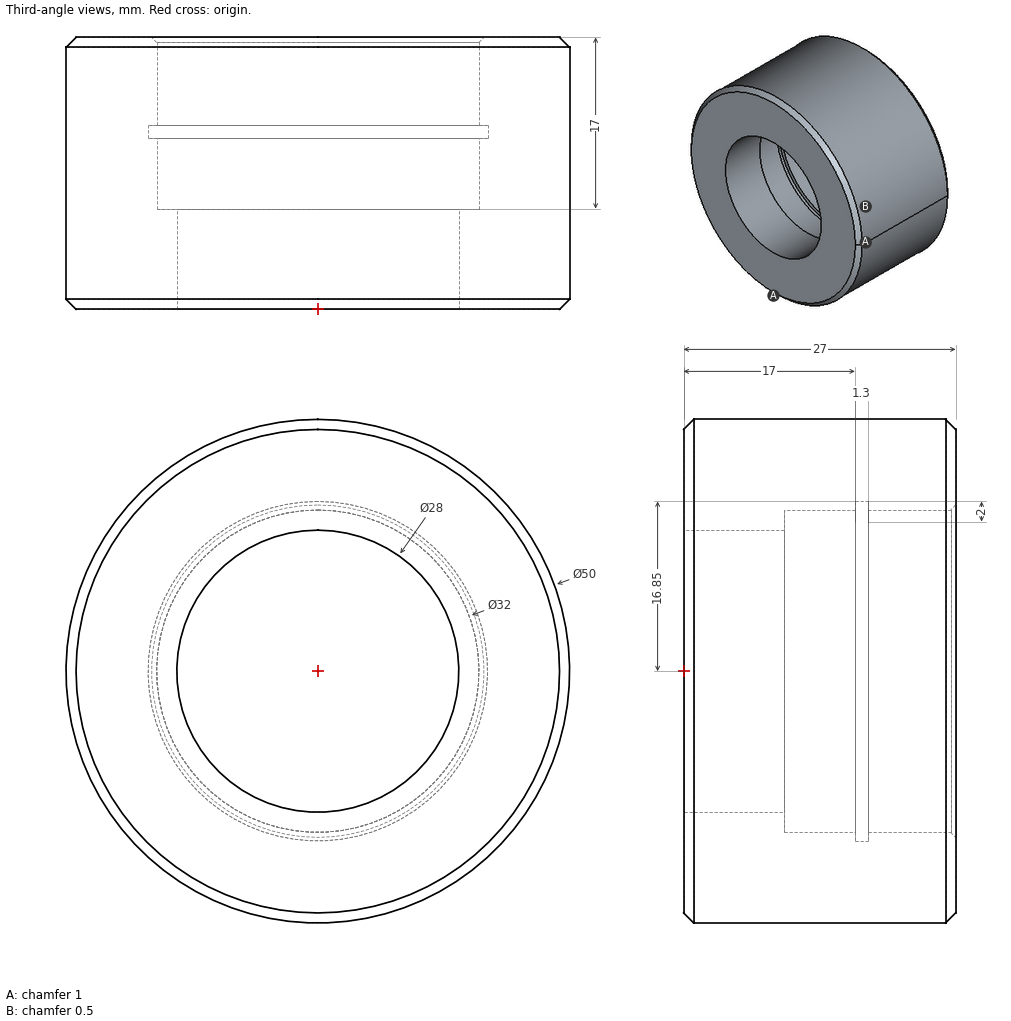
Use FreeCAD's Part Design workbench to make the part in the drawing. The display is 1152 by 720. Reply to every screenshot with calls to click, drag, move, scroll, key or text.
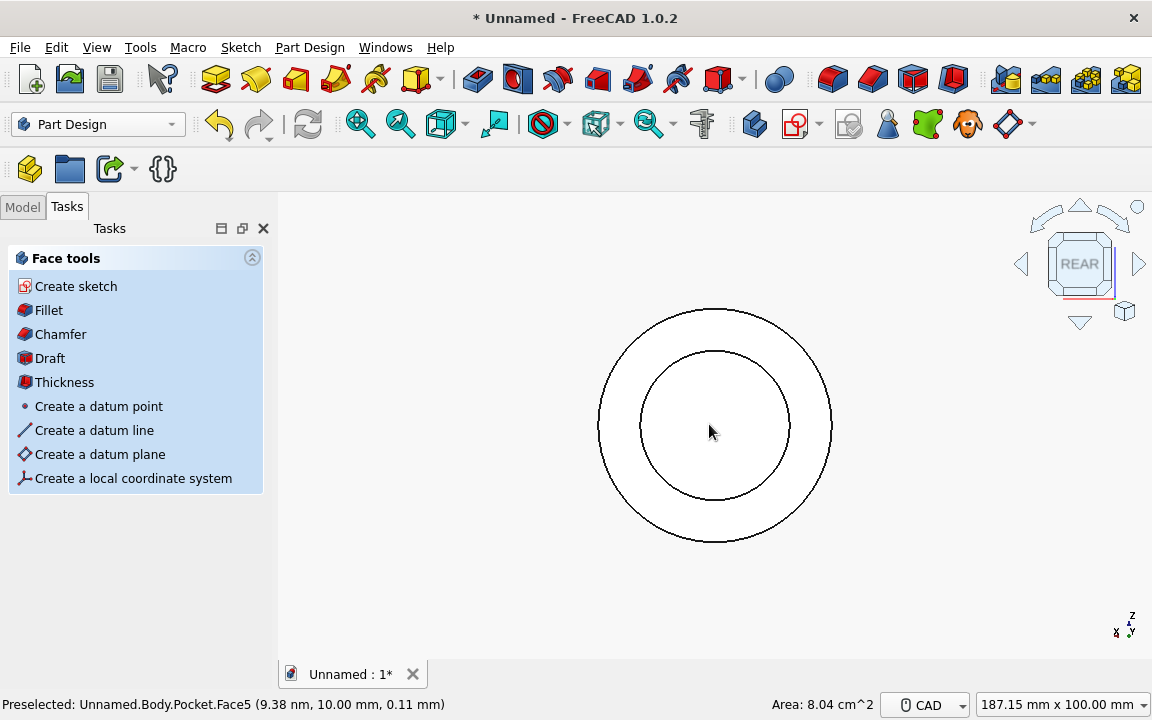
click(796, 124)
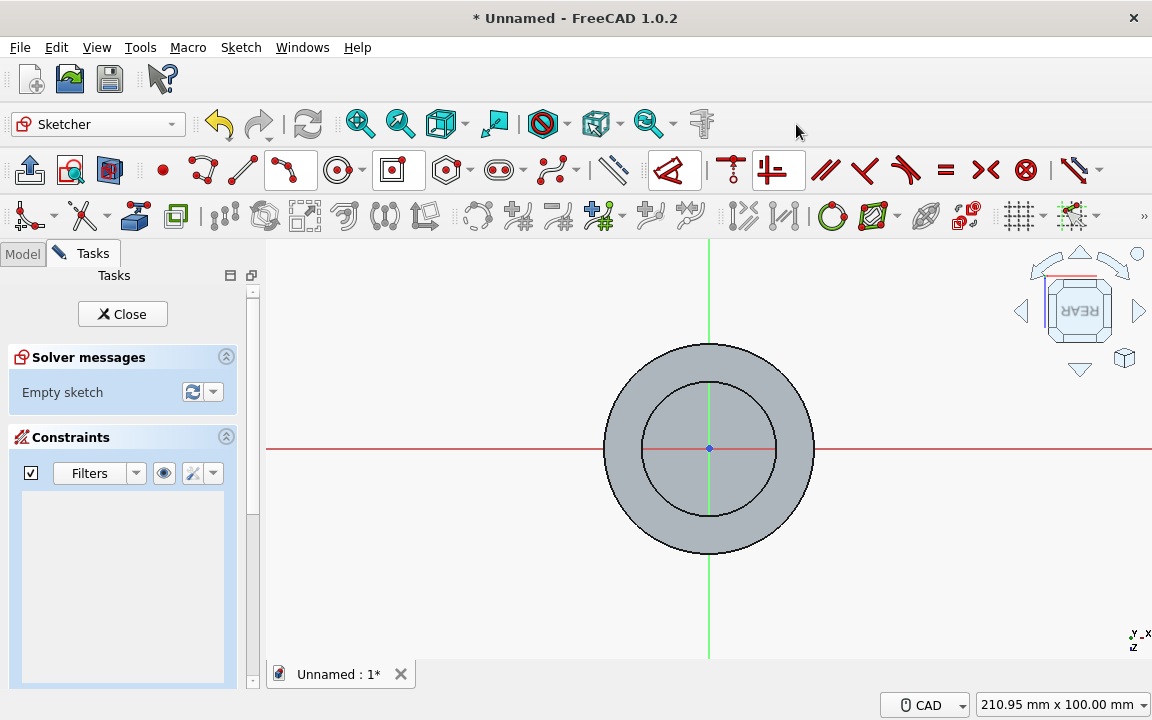
click(110, 170)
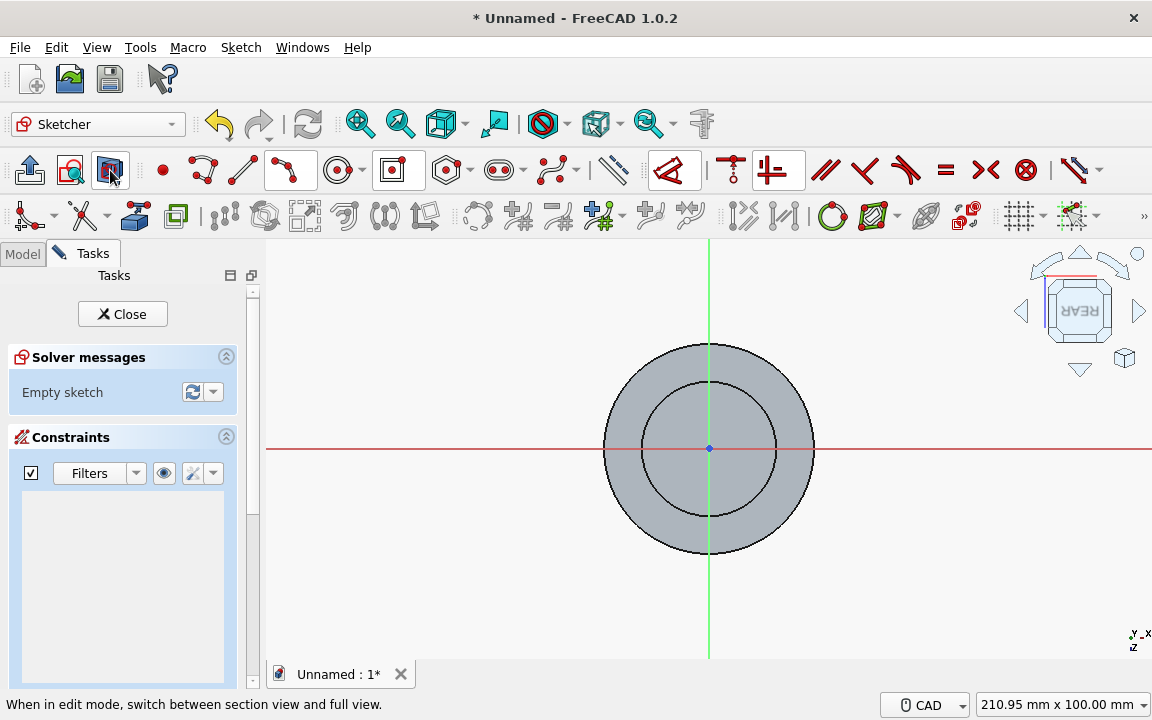
scroll(765, 449, up, 4)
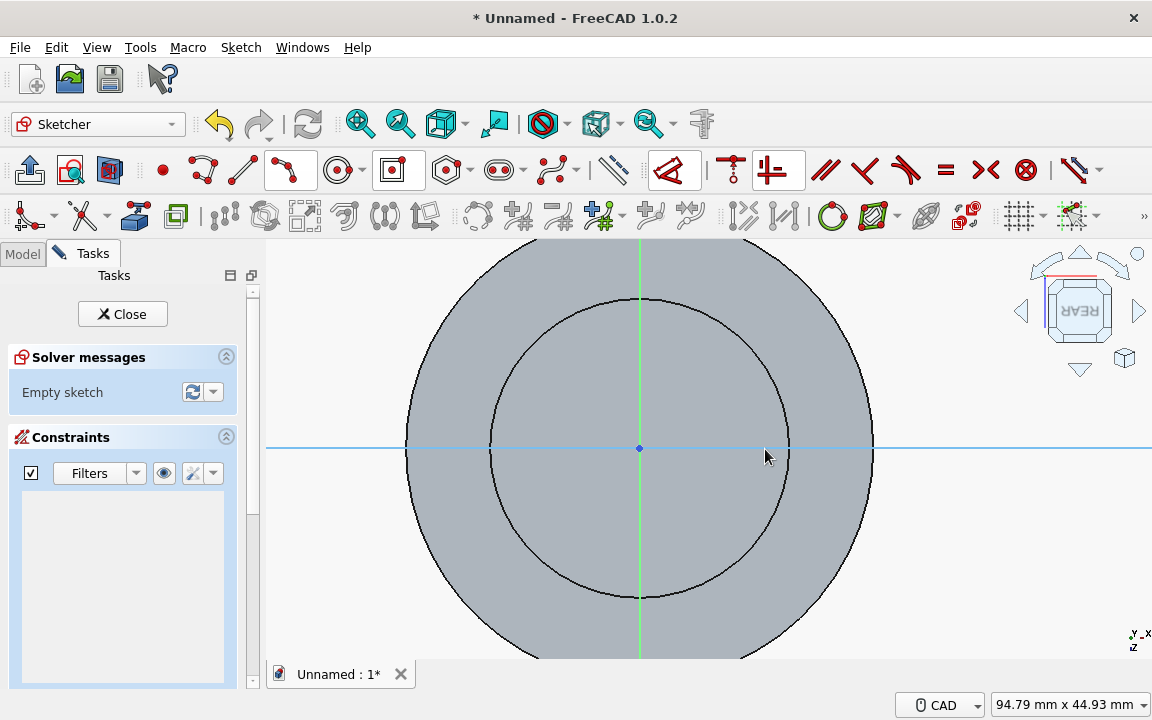
click(338, 170)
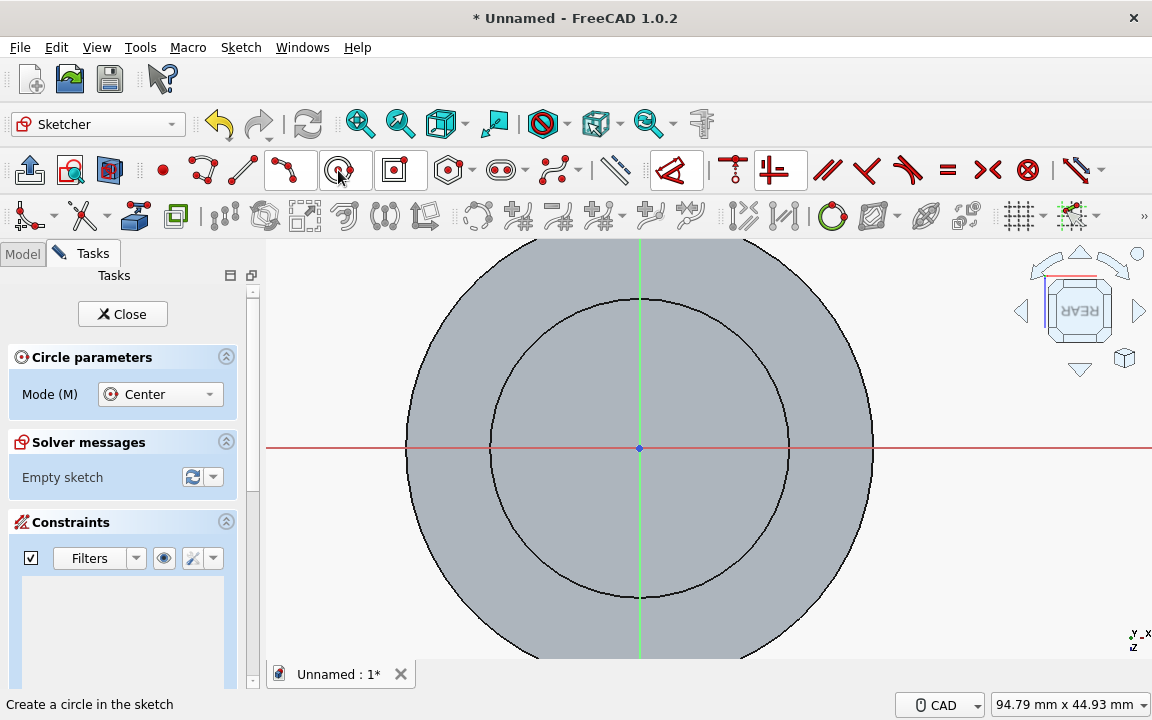
click(640, 448)
move(732, 356)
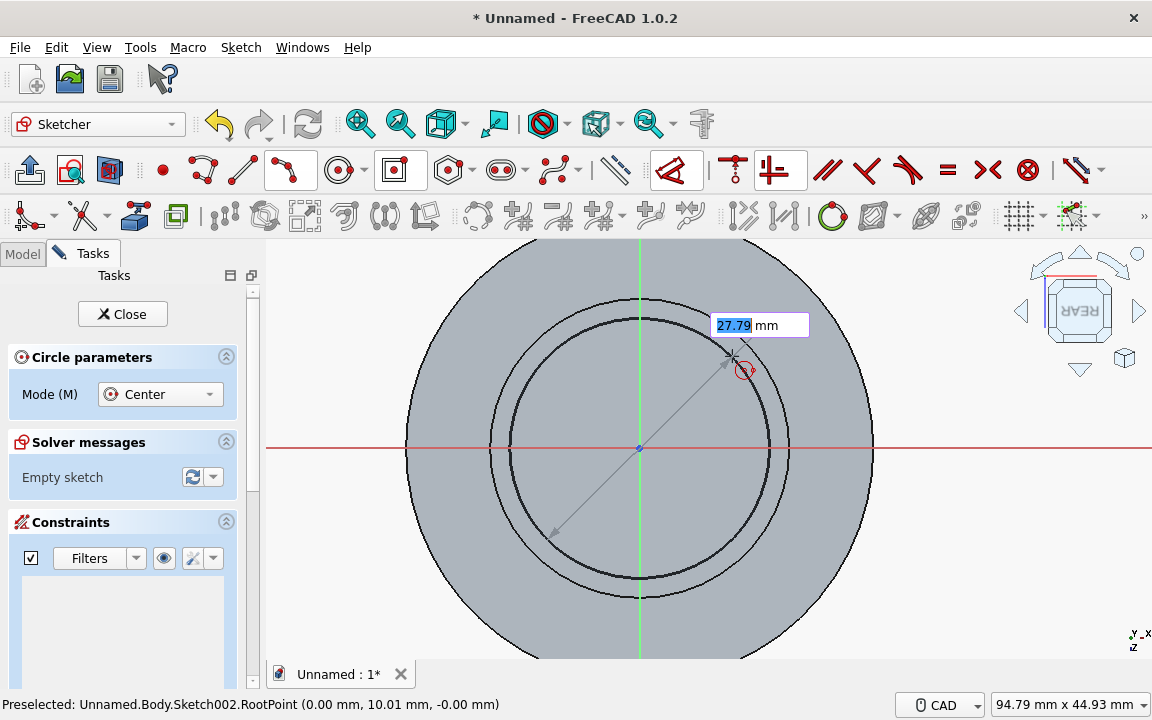
text(28)
key(Return)
key(Escape)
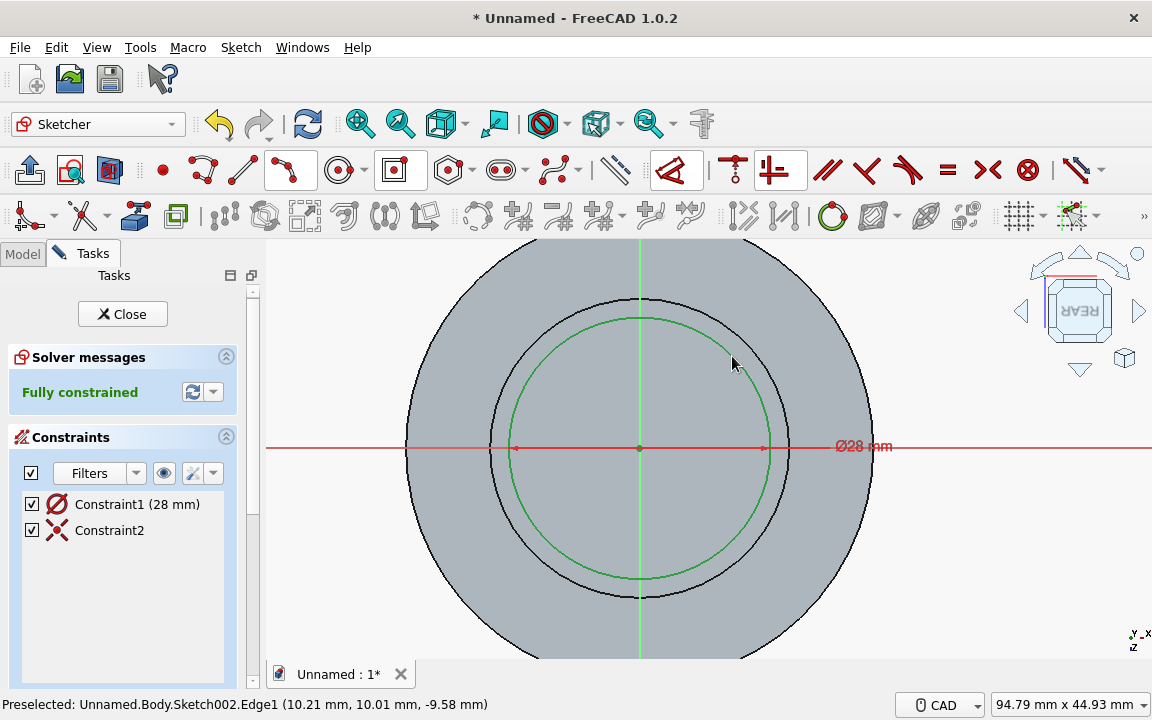
click(123, 314)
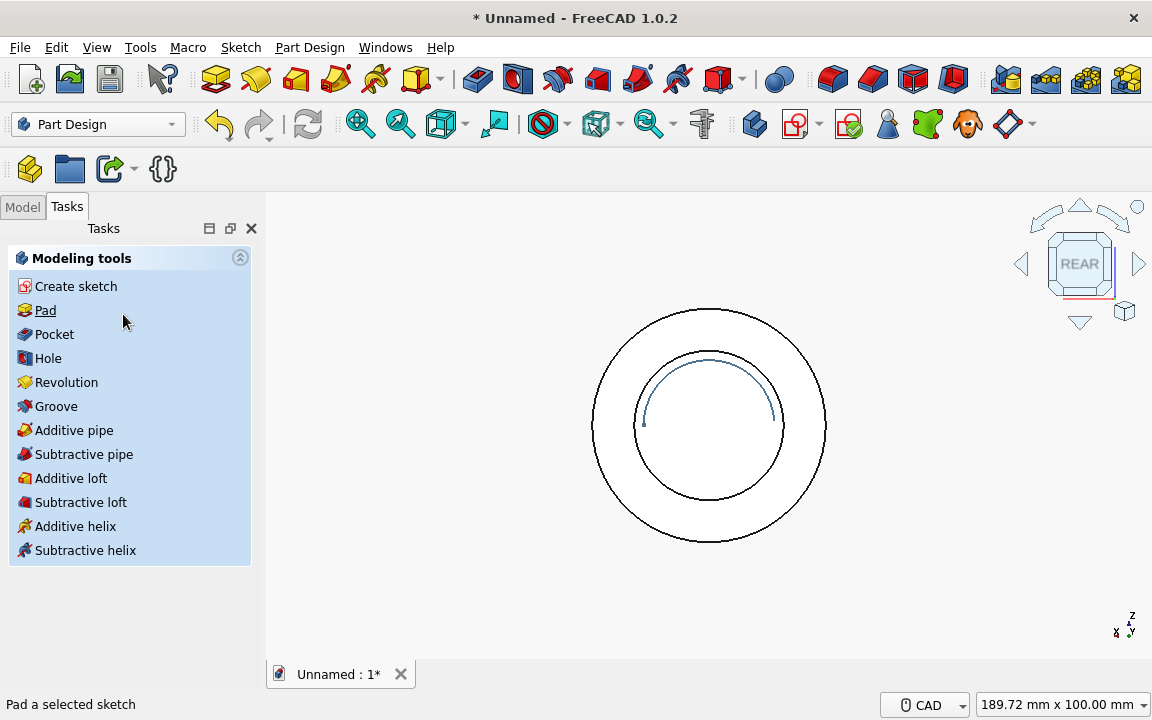
click(478, 80)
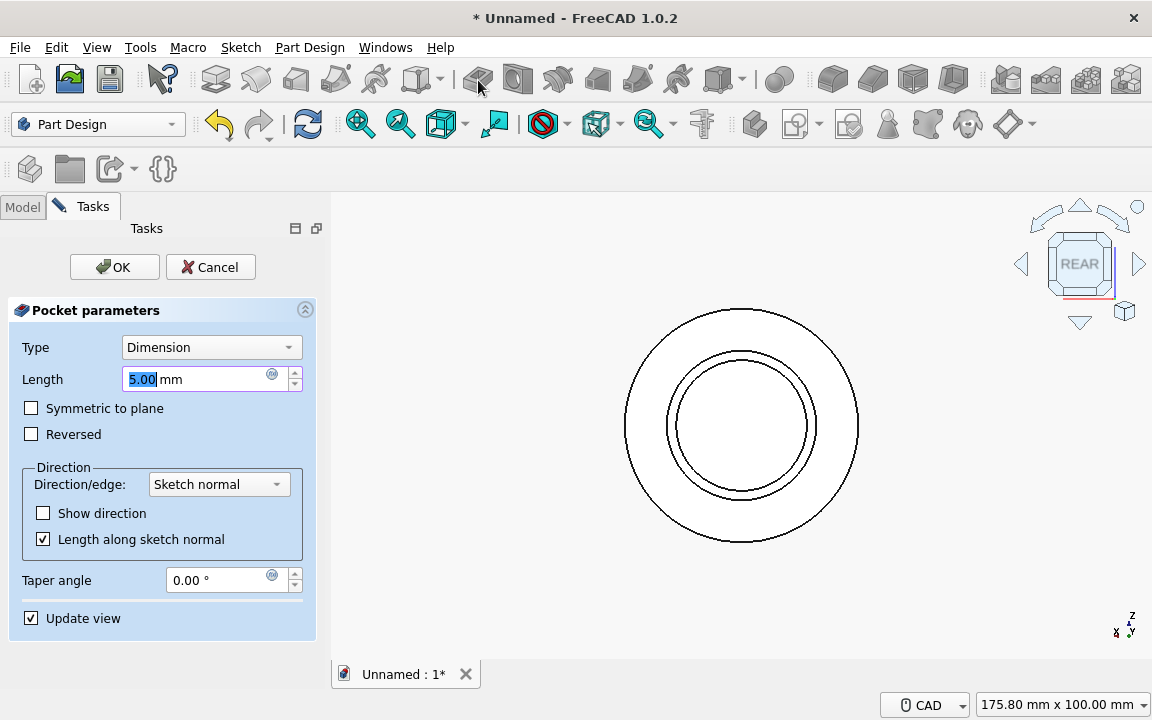
click(212, 348)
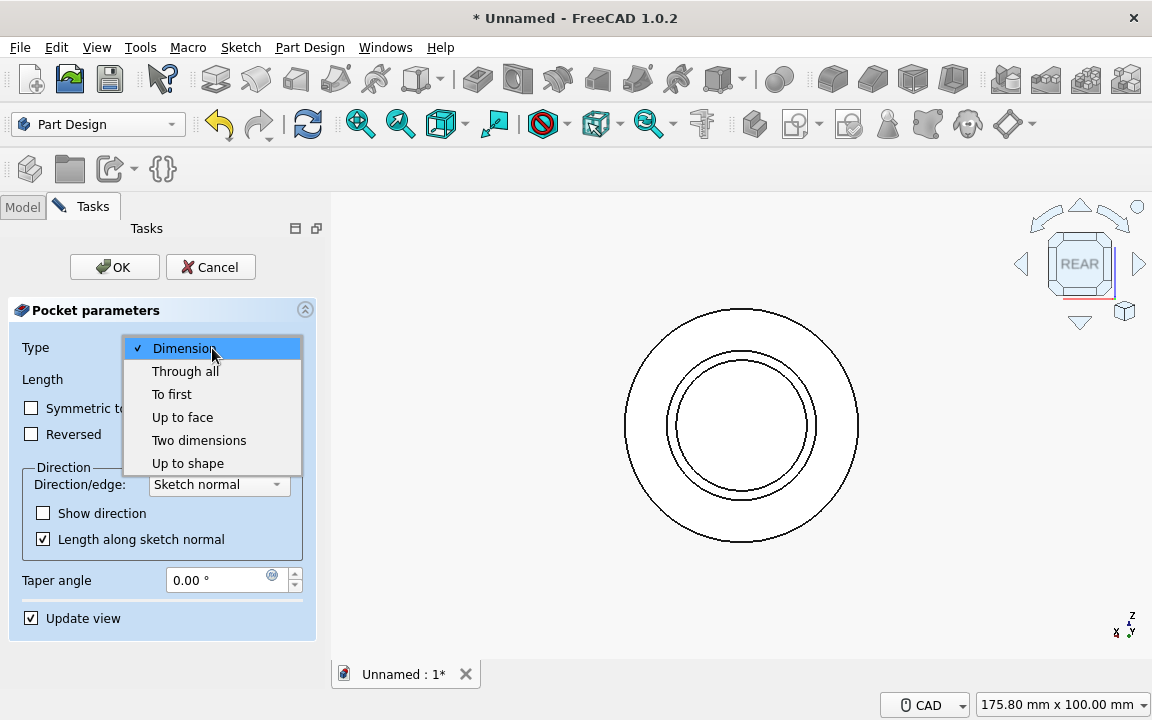
click(212, 372)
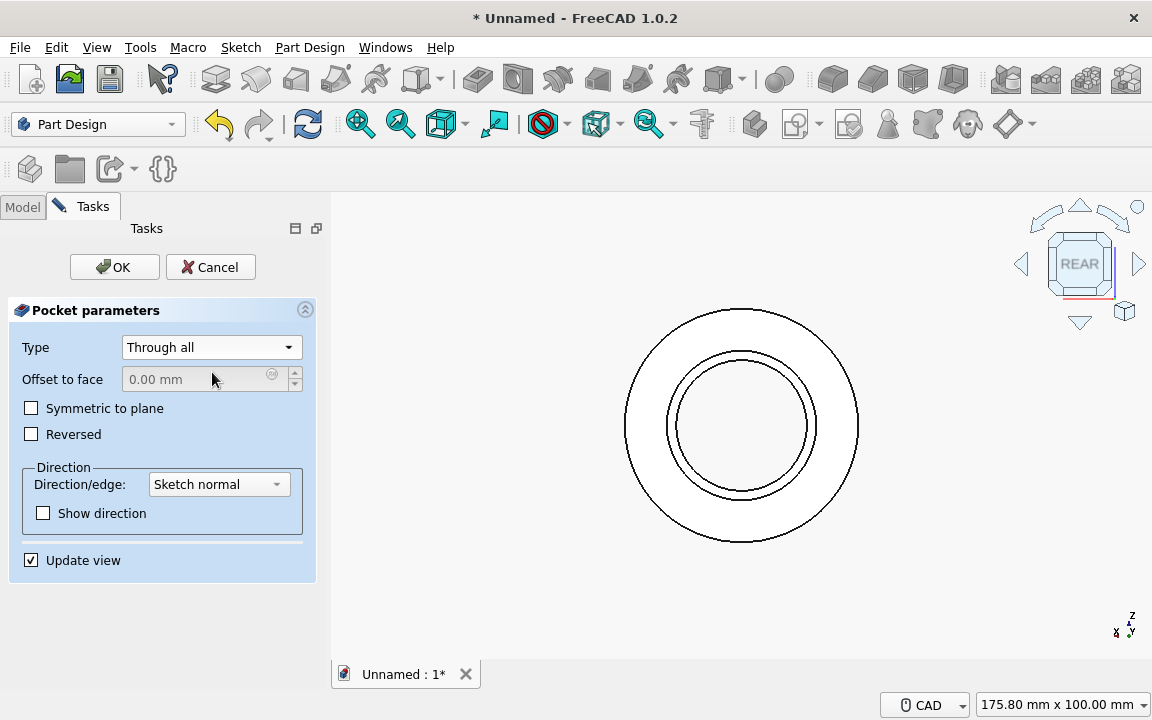
click(115, 267)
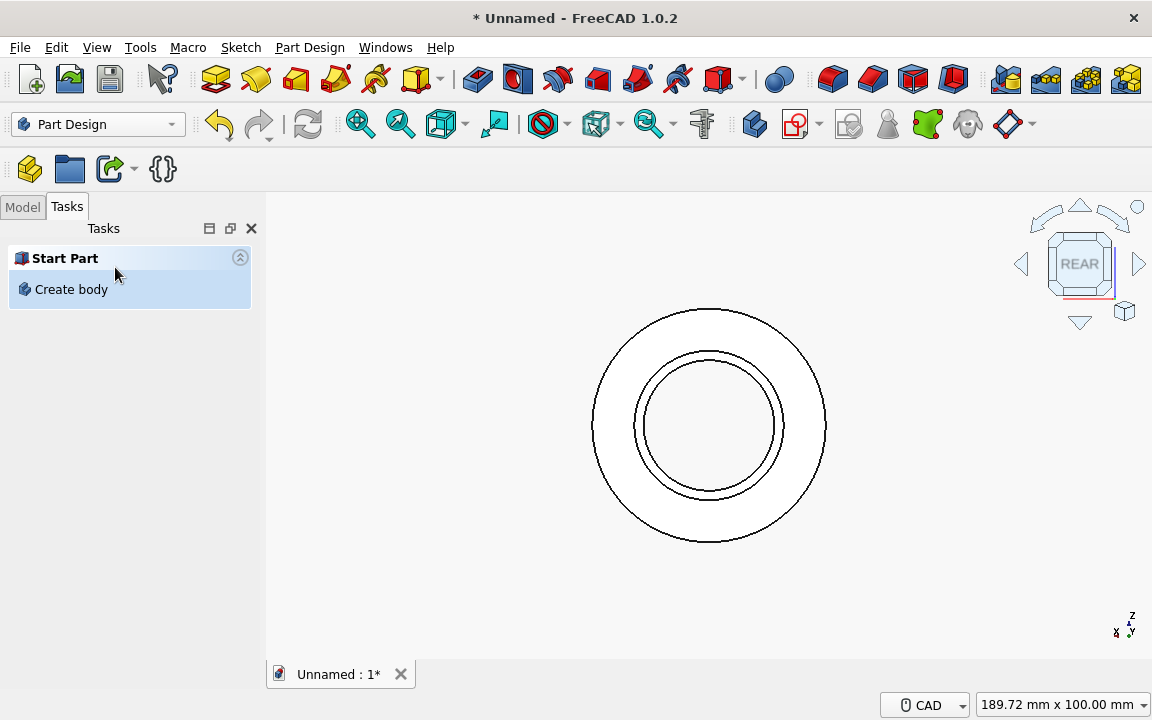
click(826, 425)